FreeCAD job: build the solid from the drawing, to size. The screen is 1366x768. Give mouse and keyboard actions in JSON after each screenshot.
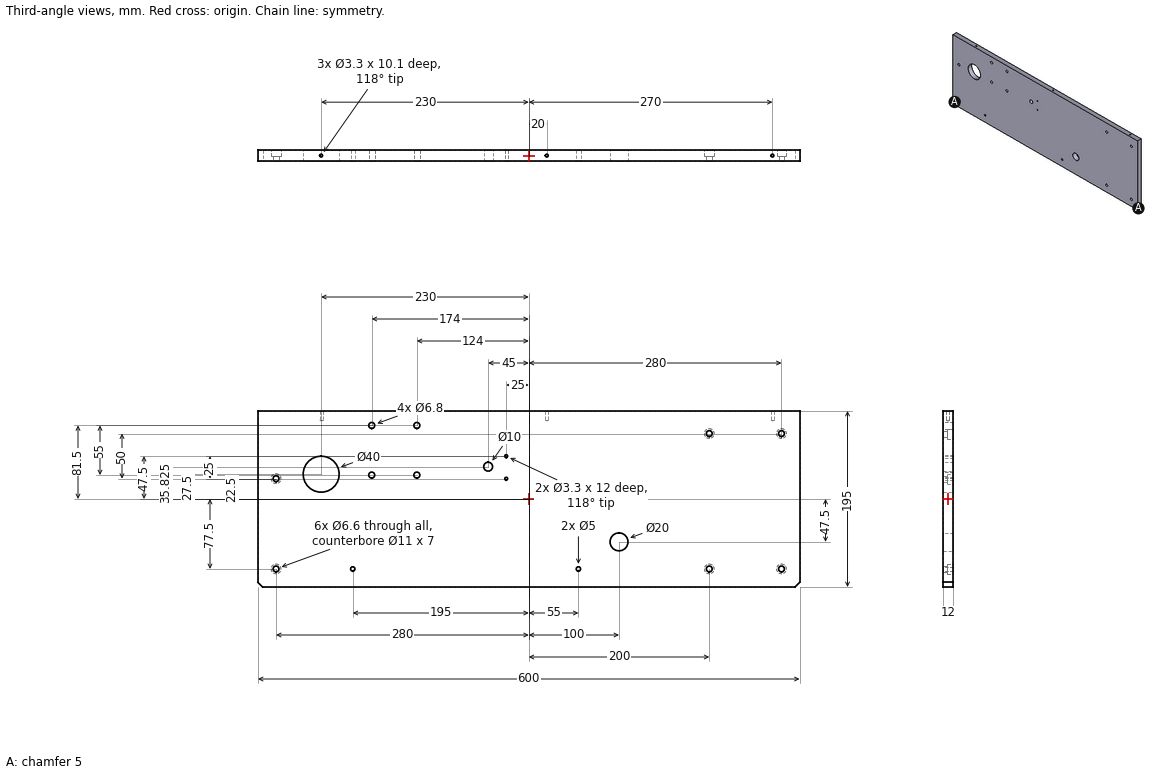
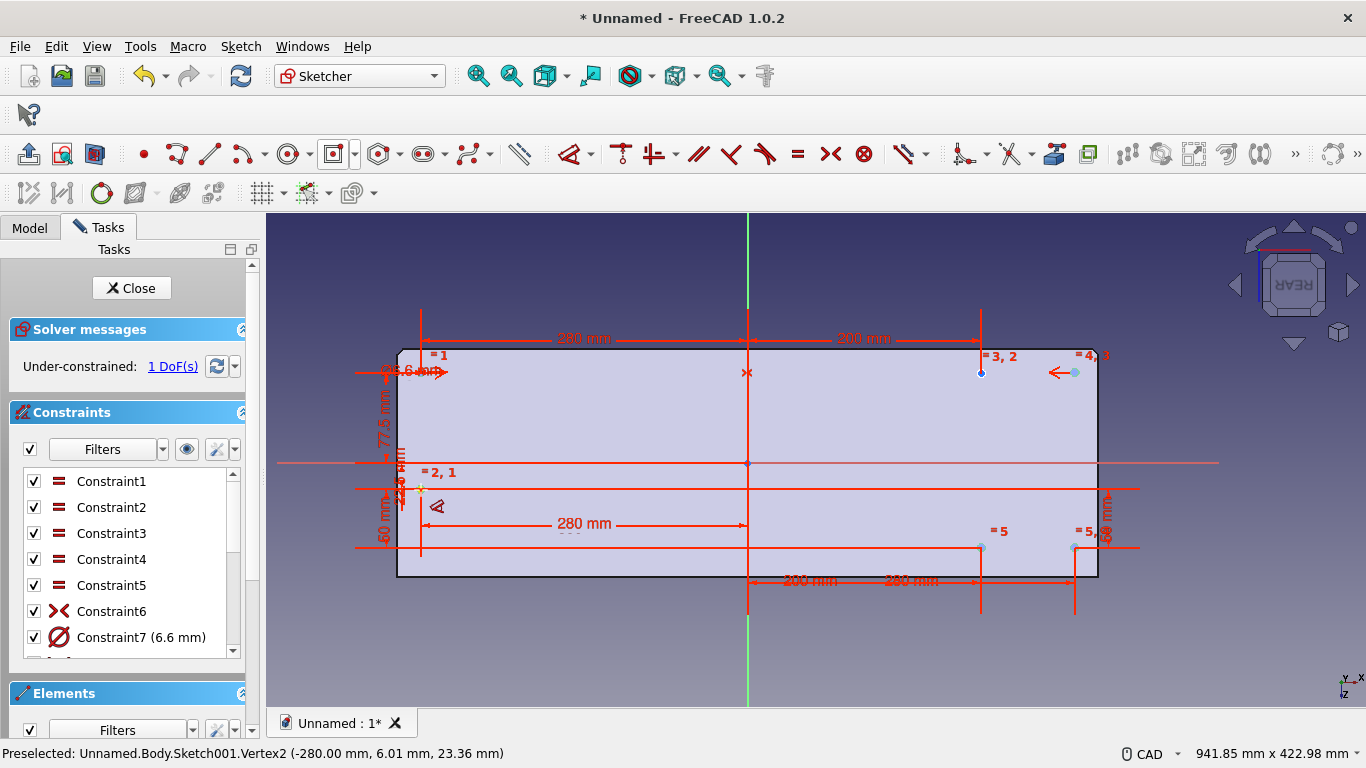
{"action": "left_click", "coordinate": [981, 374]}
{"action": "left_click", "coordinate": [1015, 418]}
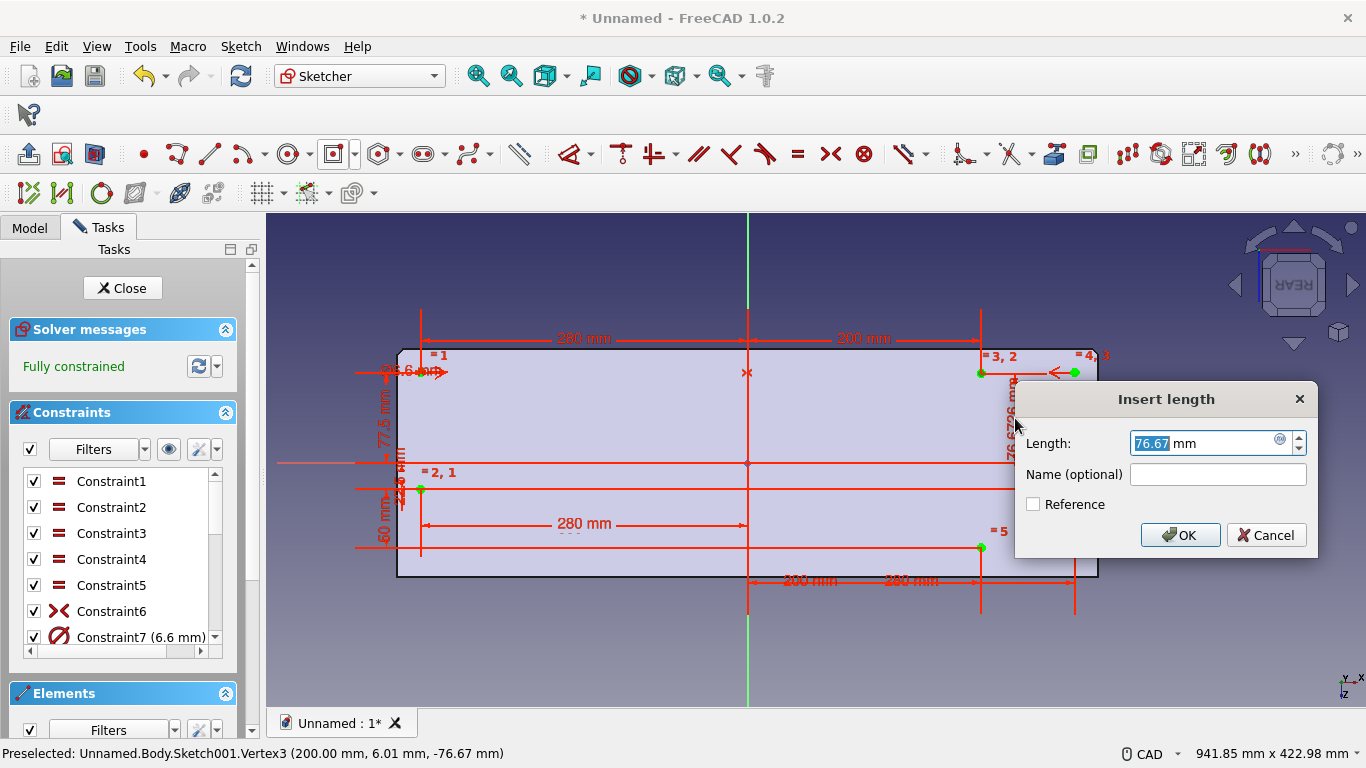
{"action": "type", "text": "77.5"}
{"action": "key", "text": "Return"}
{"action": "key", "text": "Escape"}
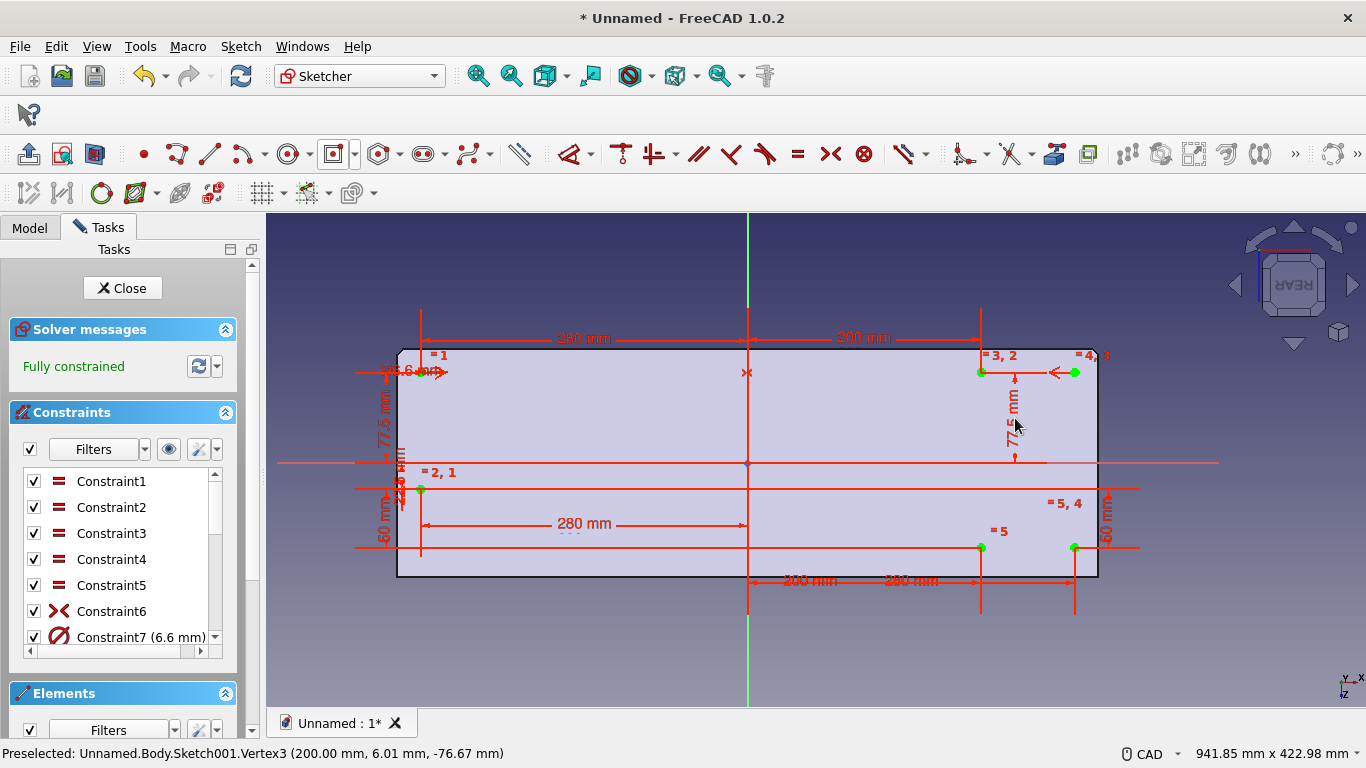
{"action": "left_click", "coordinate": [123, 288]}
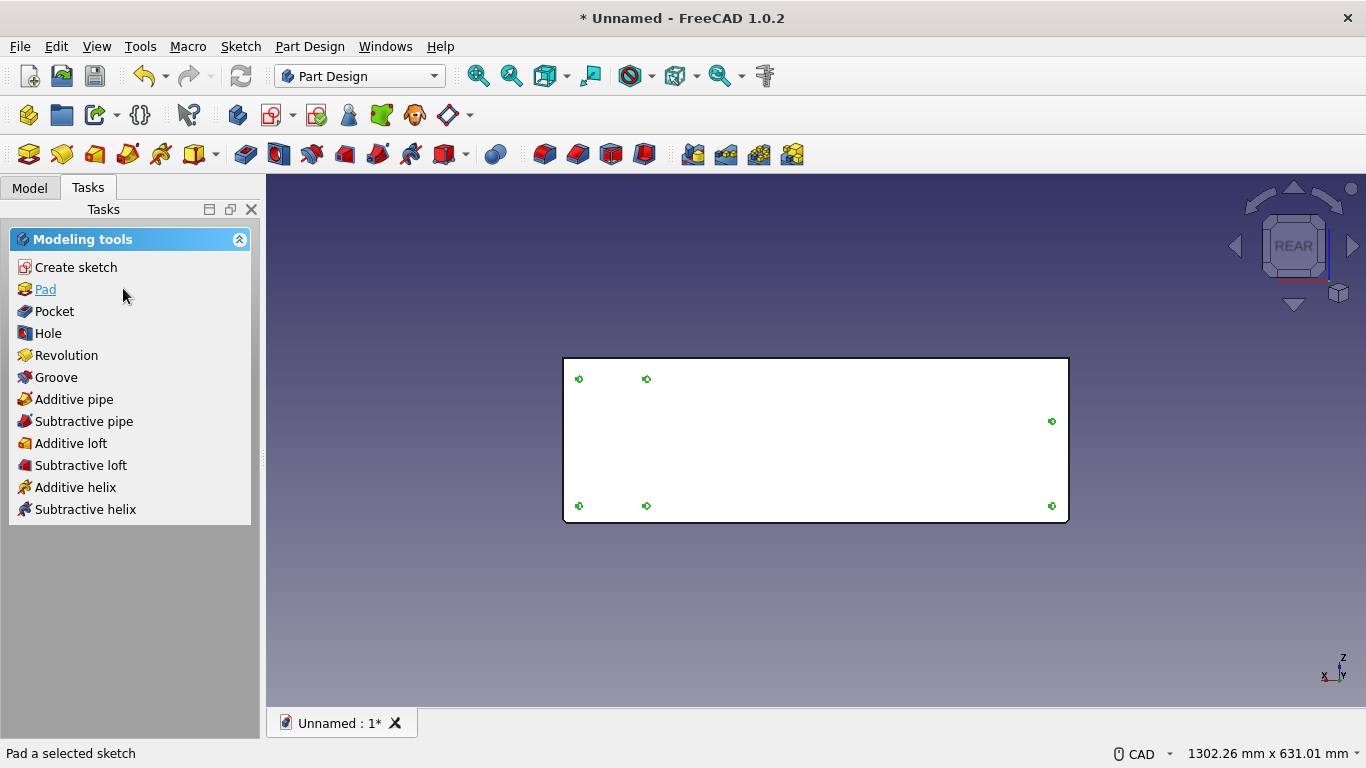
{"action": "left_click", "coordinate": [279, 154]}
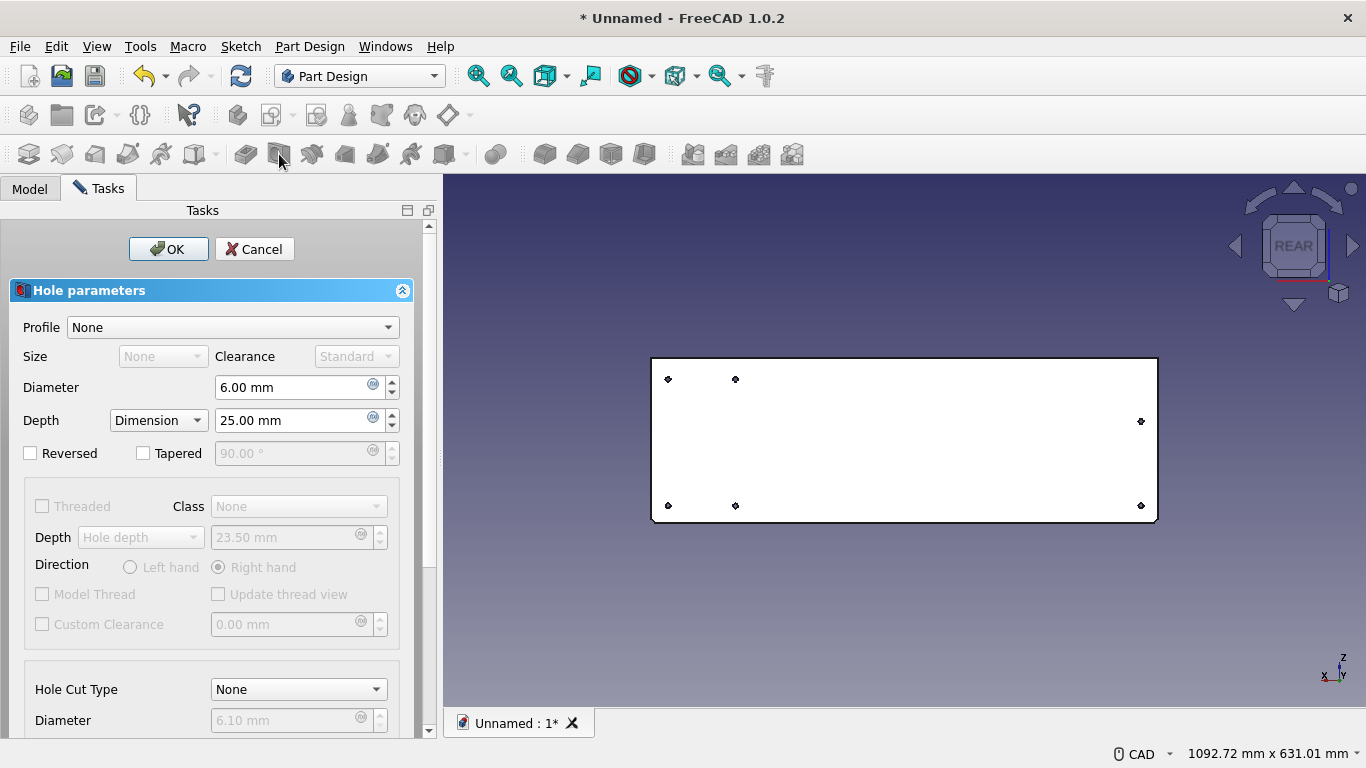
{"action": "triple_click", "coordinate": [300, 388]}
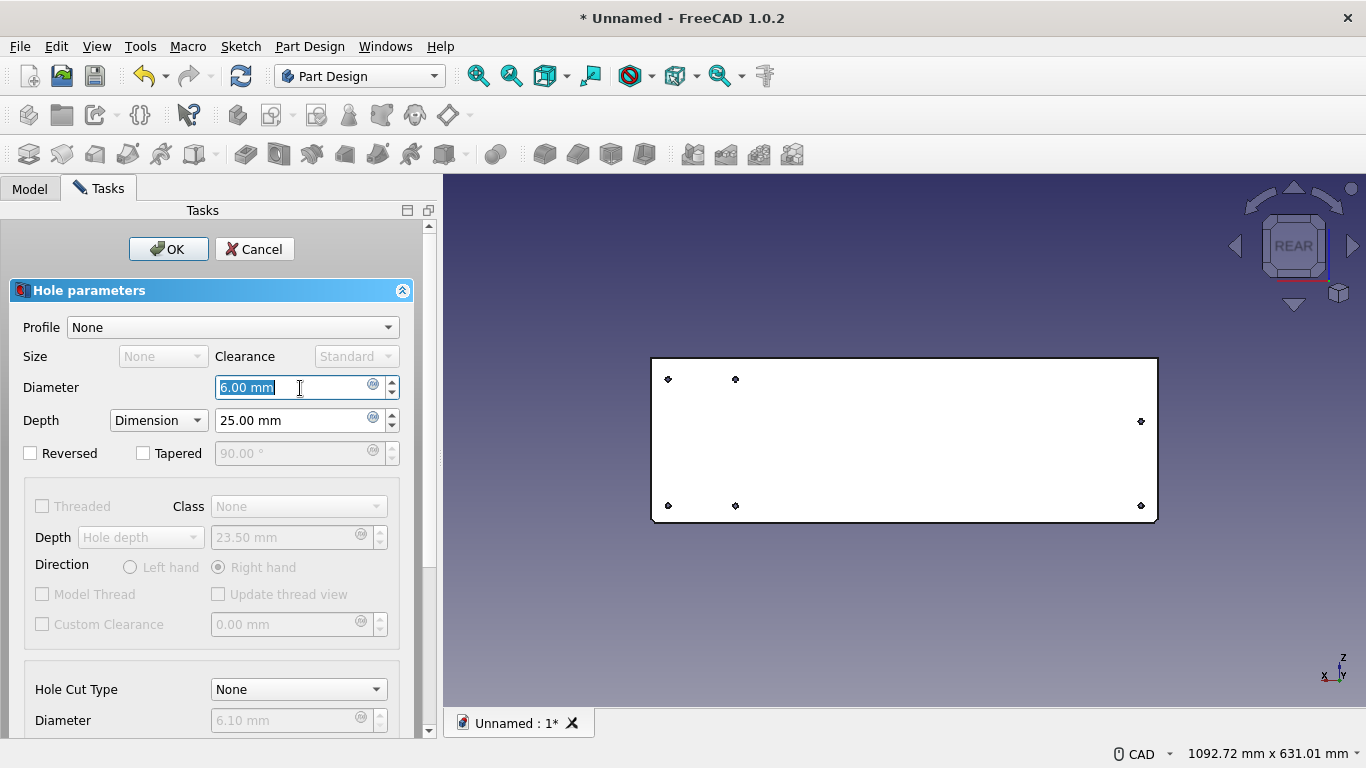
{"action": "type", "text": "6.6"}
{"action": "key", "text": "Tab"}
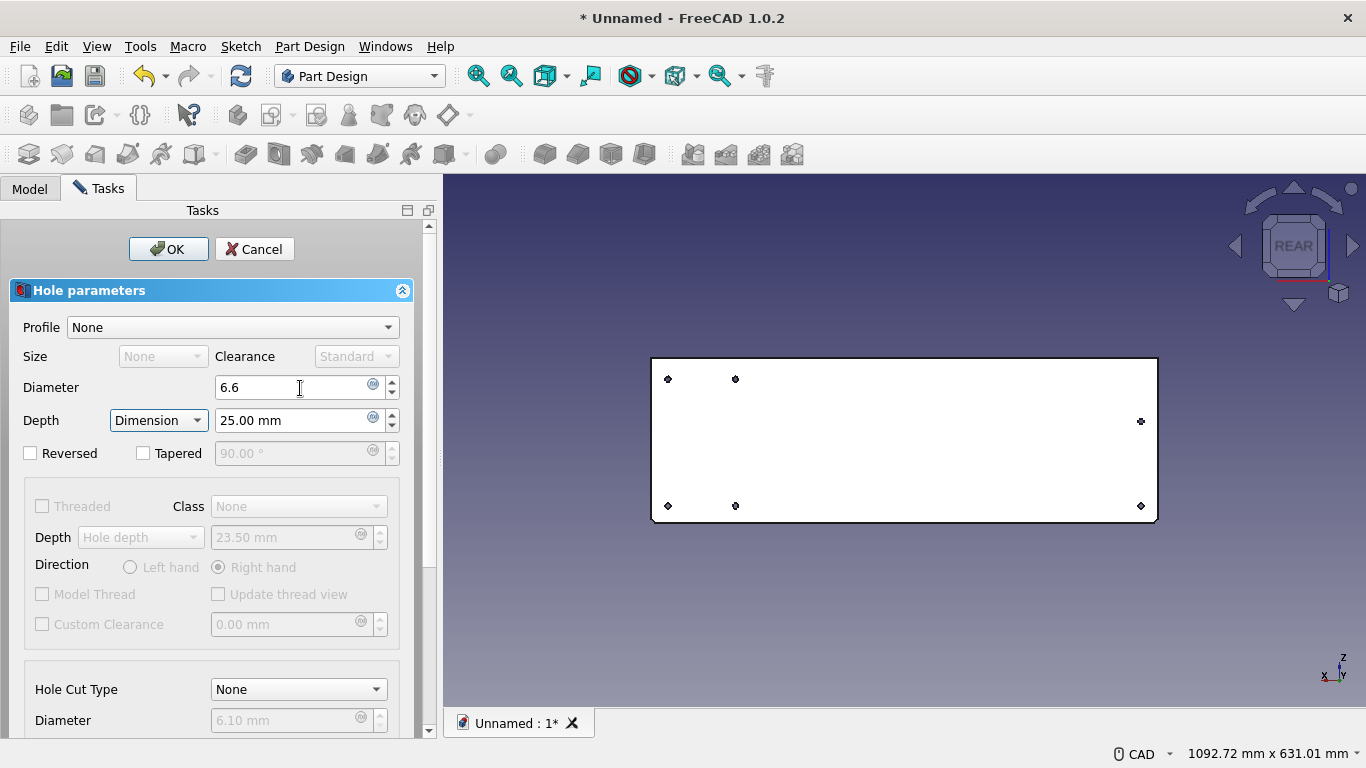
{"action": "left_click", "coordinate": [160, 420]}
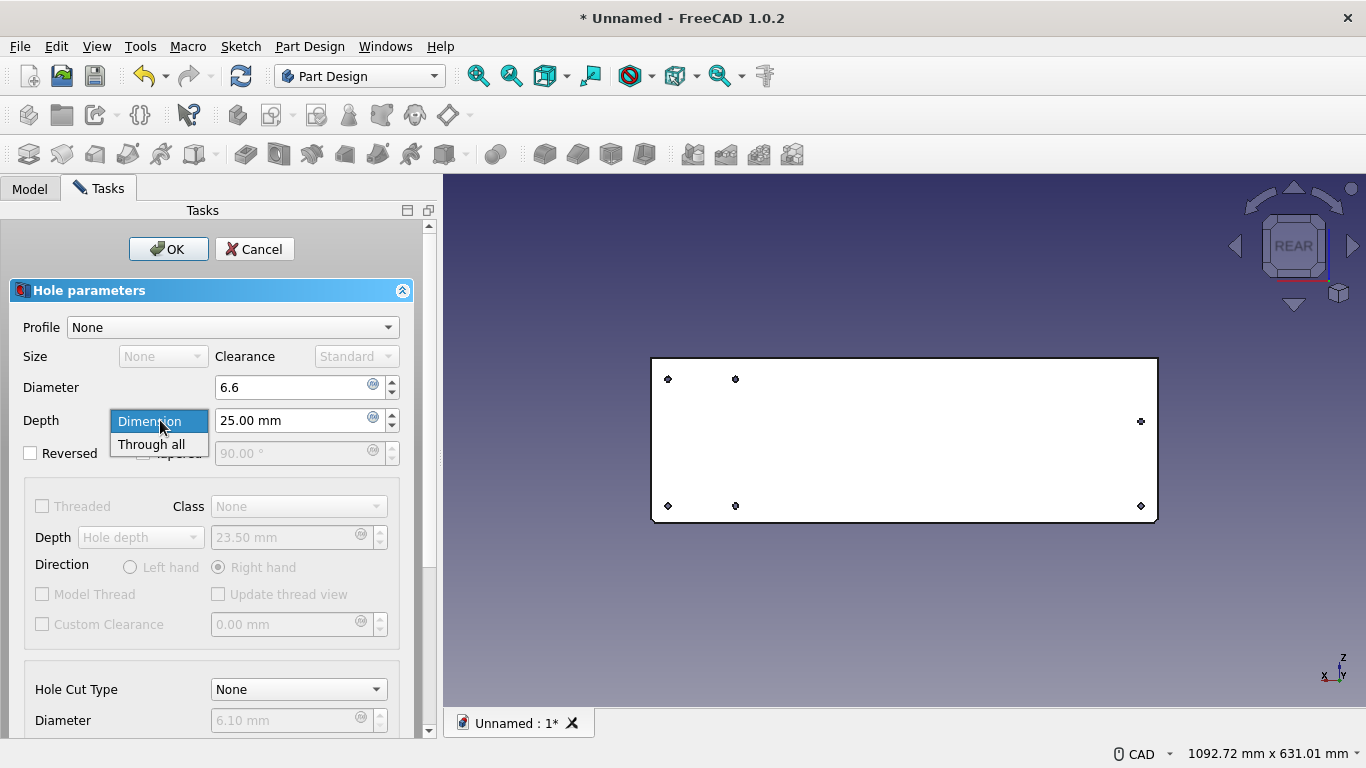
{"action": "left_click", "coordinate": [158, 444]}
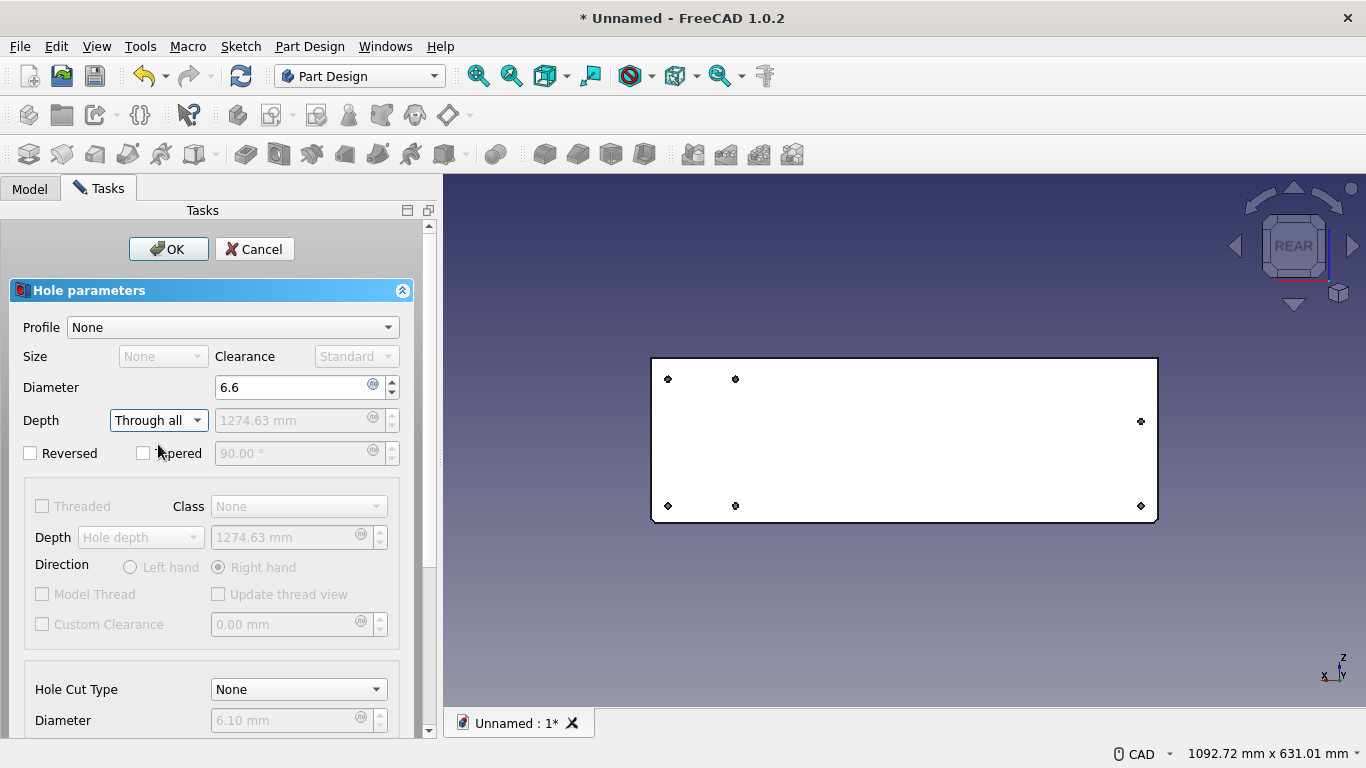
{"action": "left_click", "coordinate": [300, 690]}